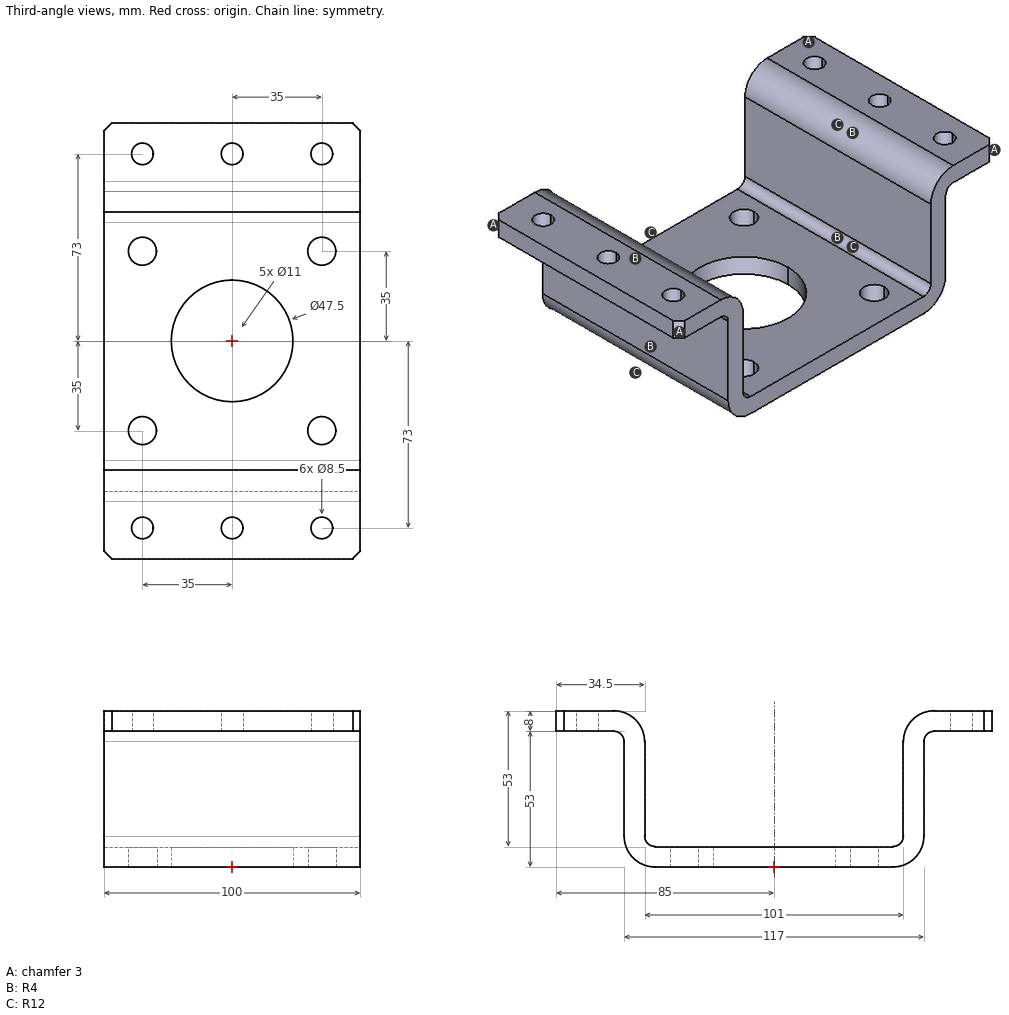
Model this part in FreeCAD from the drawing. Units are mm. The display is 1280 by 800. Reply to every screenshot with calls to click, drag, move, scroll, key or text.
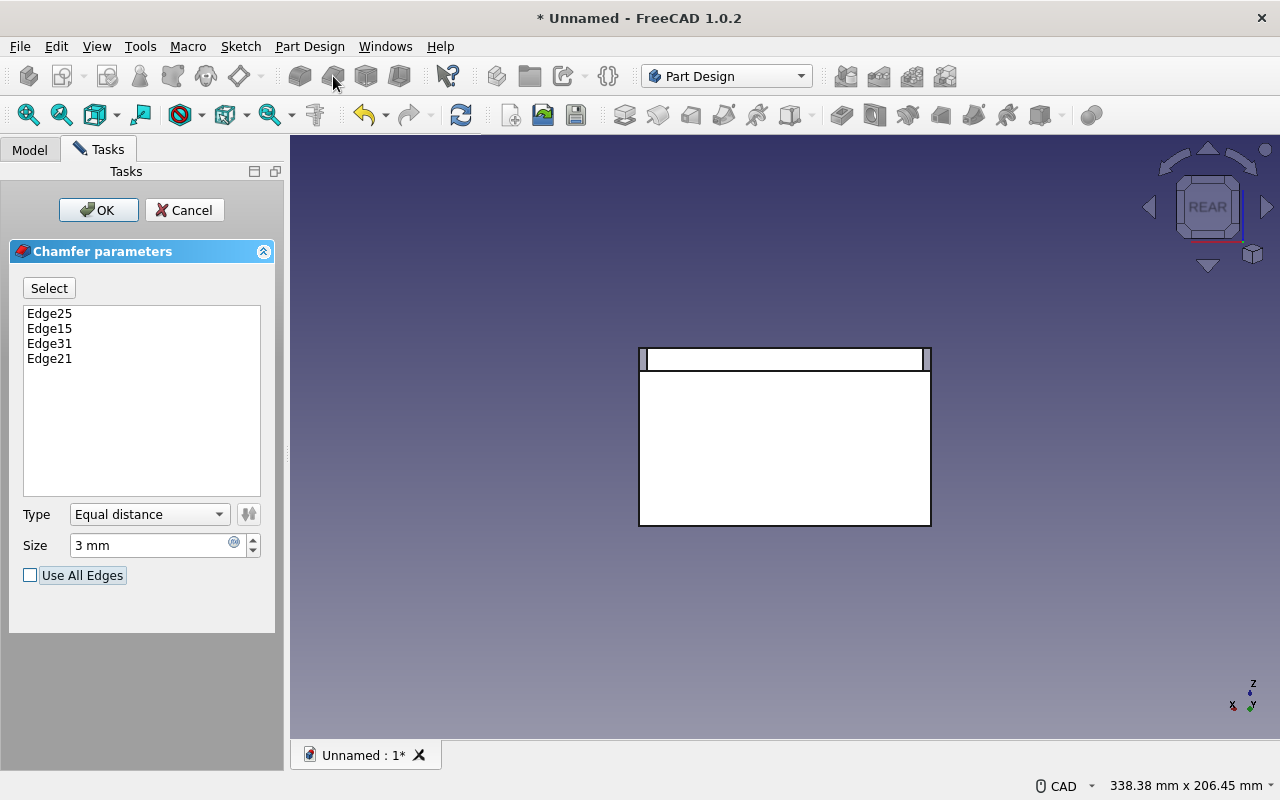
click(99, 210)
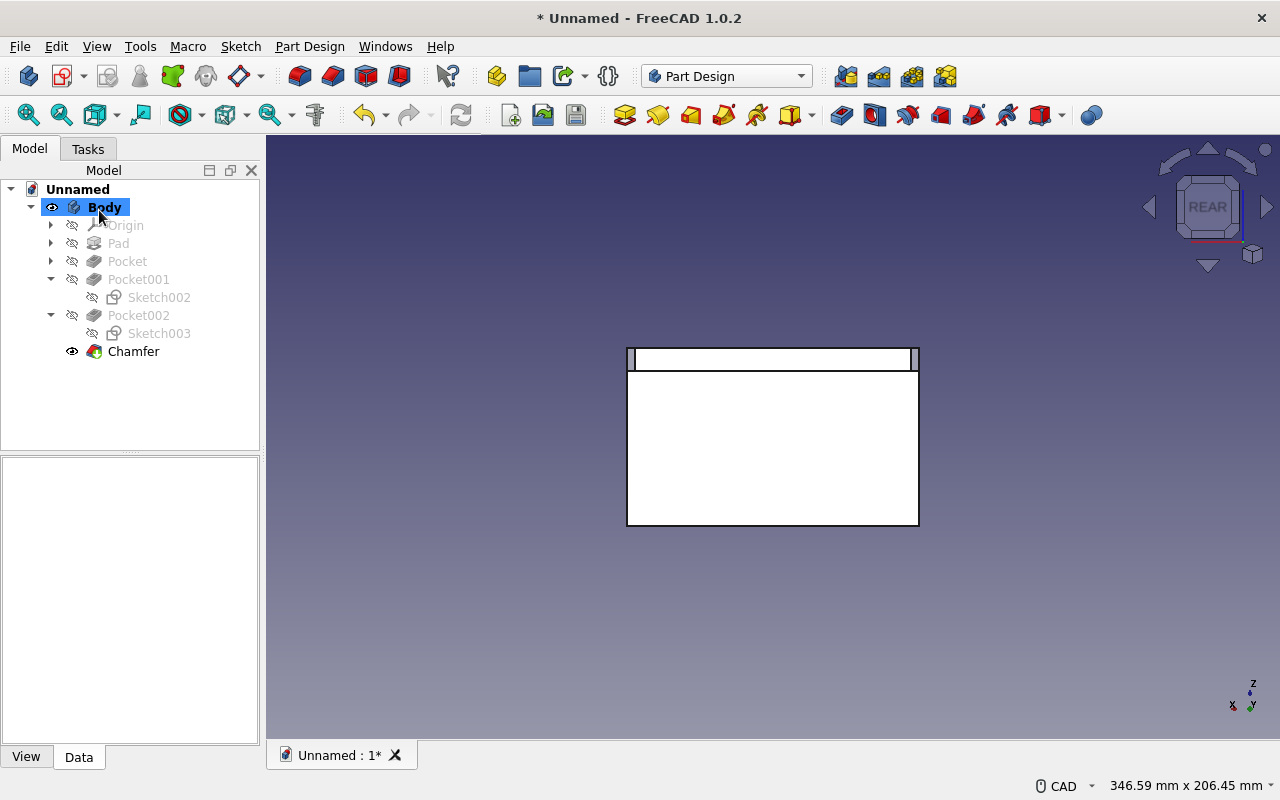
click(29, 116)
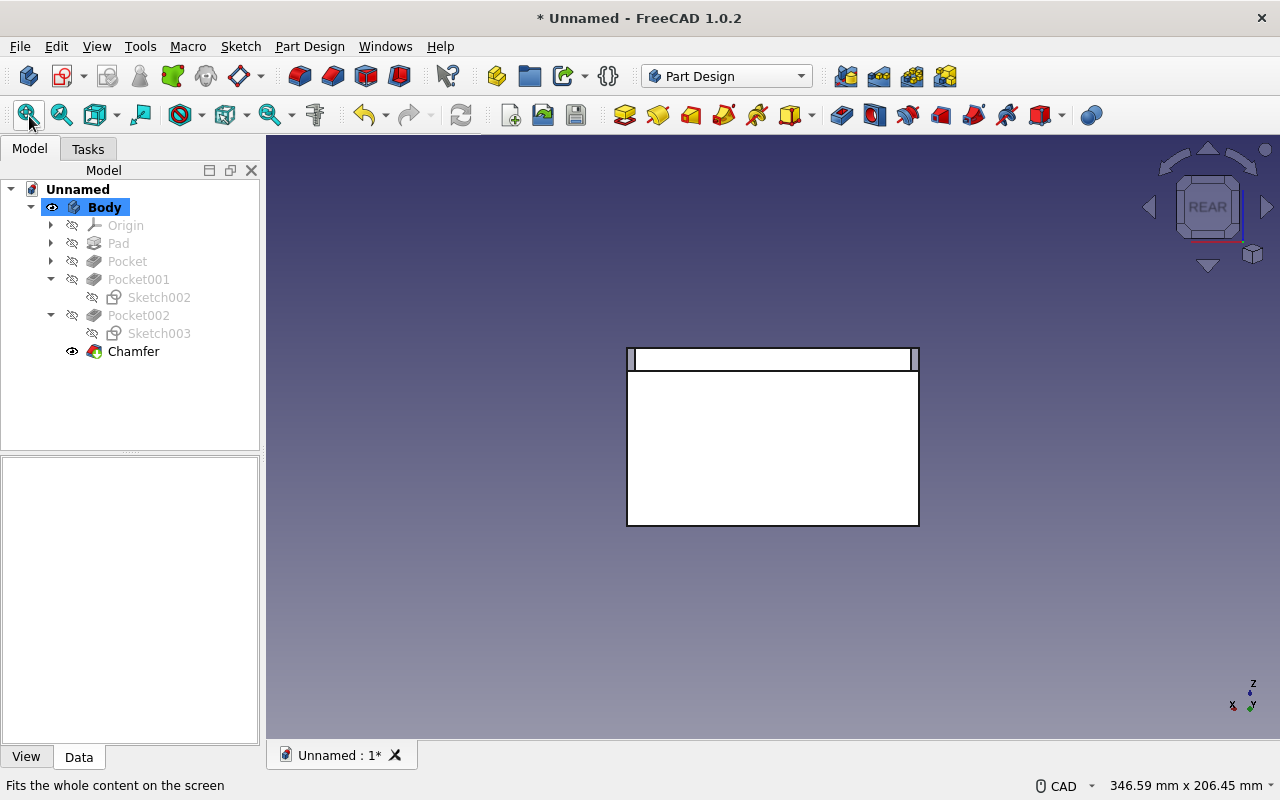
key(0)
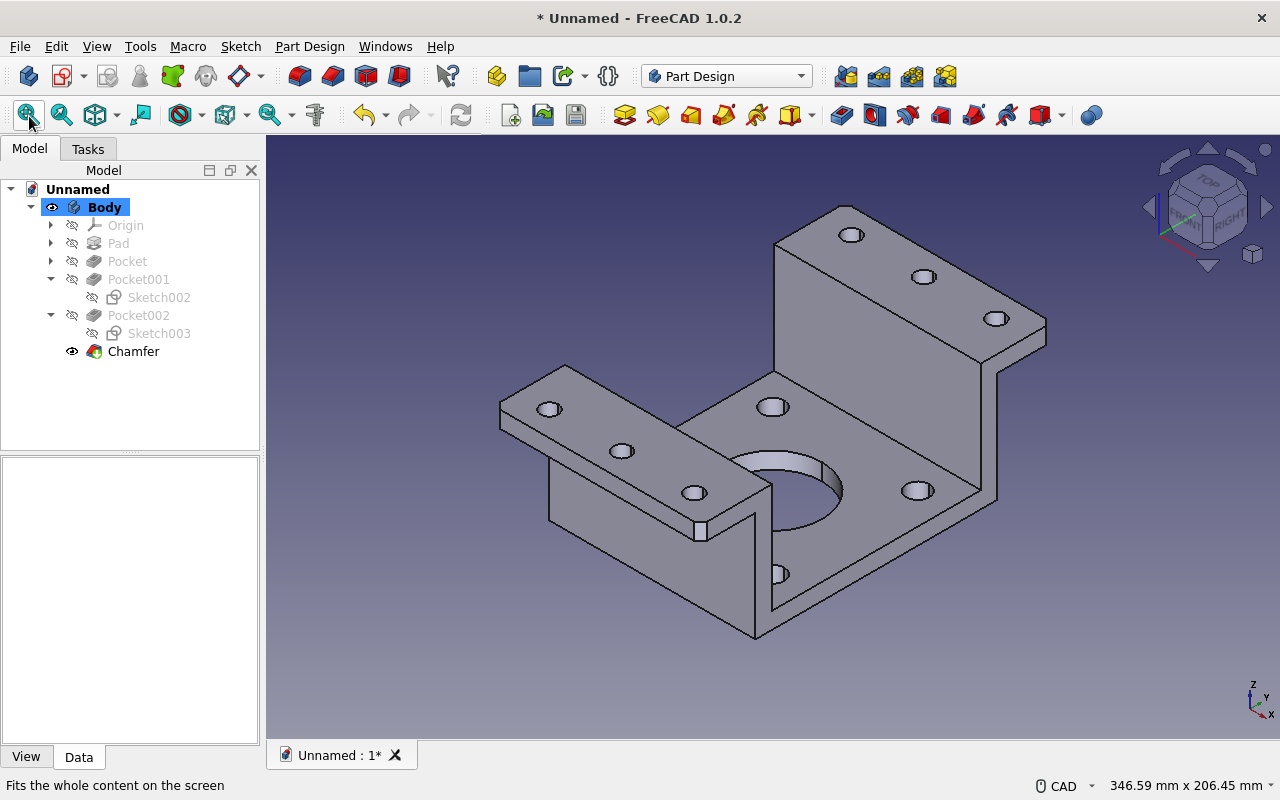
key(2)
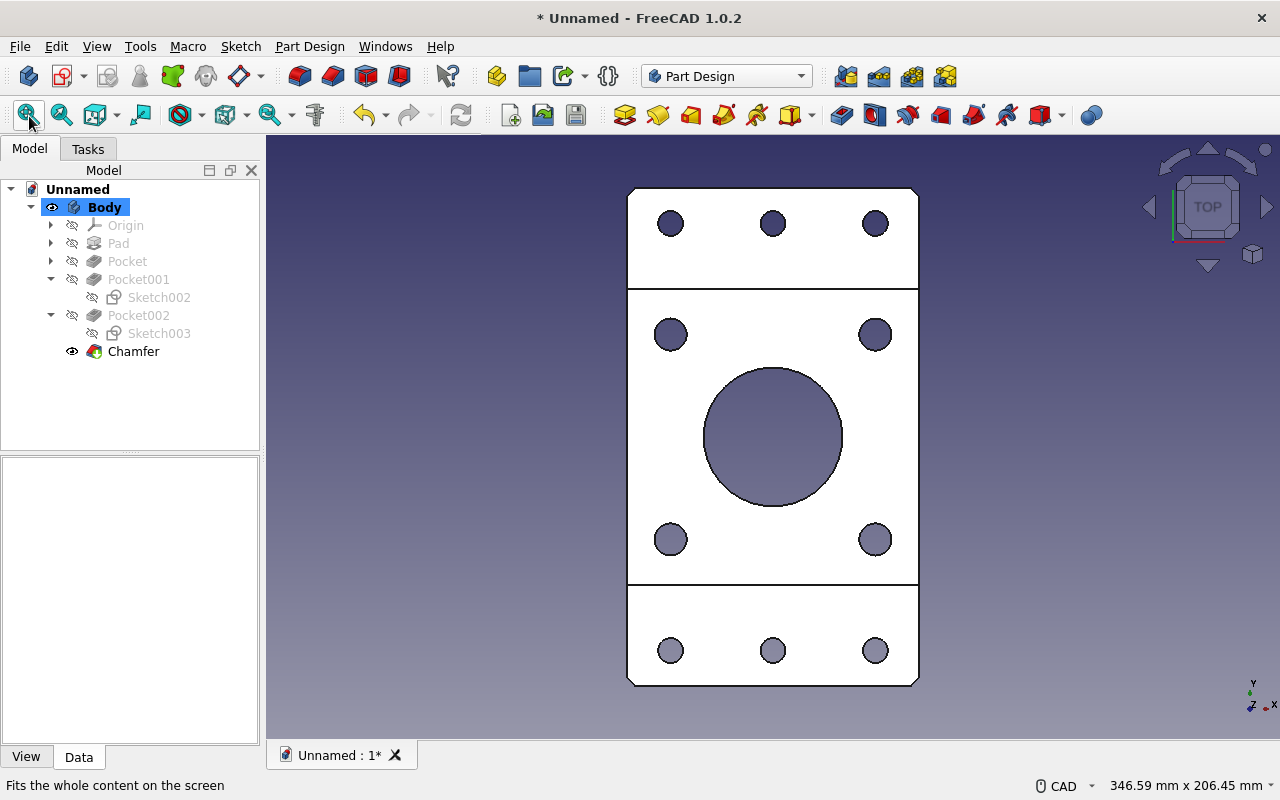
key(1)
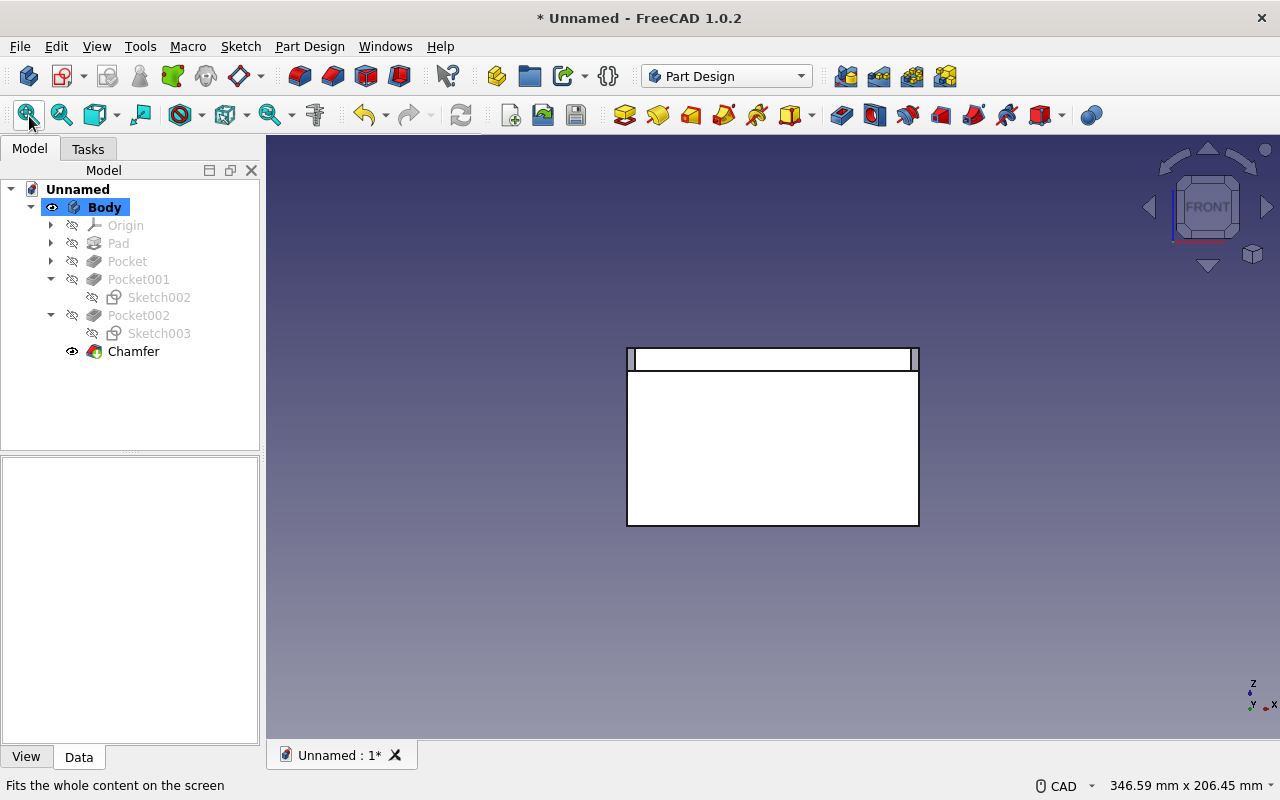
key(v)
key(f)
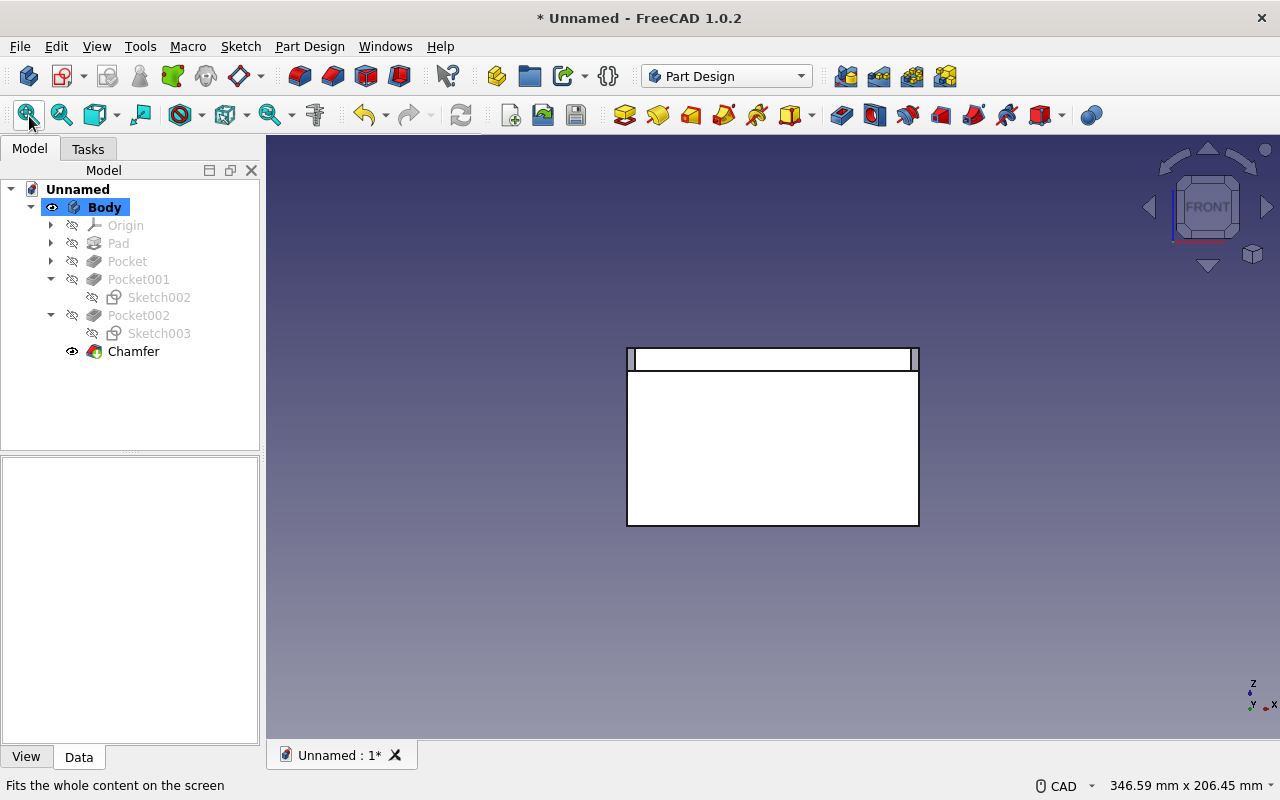
key(3)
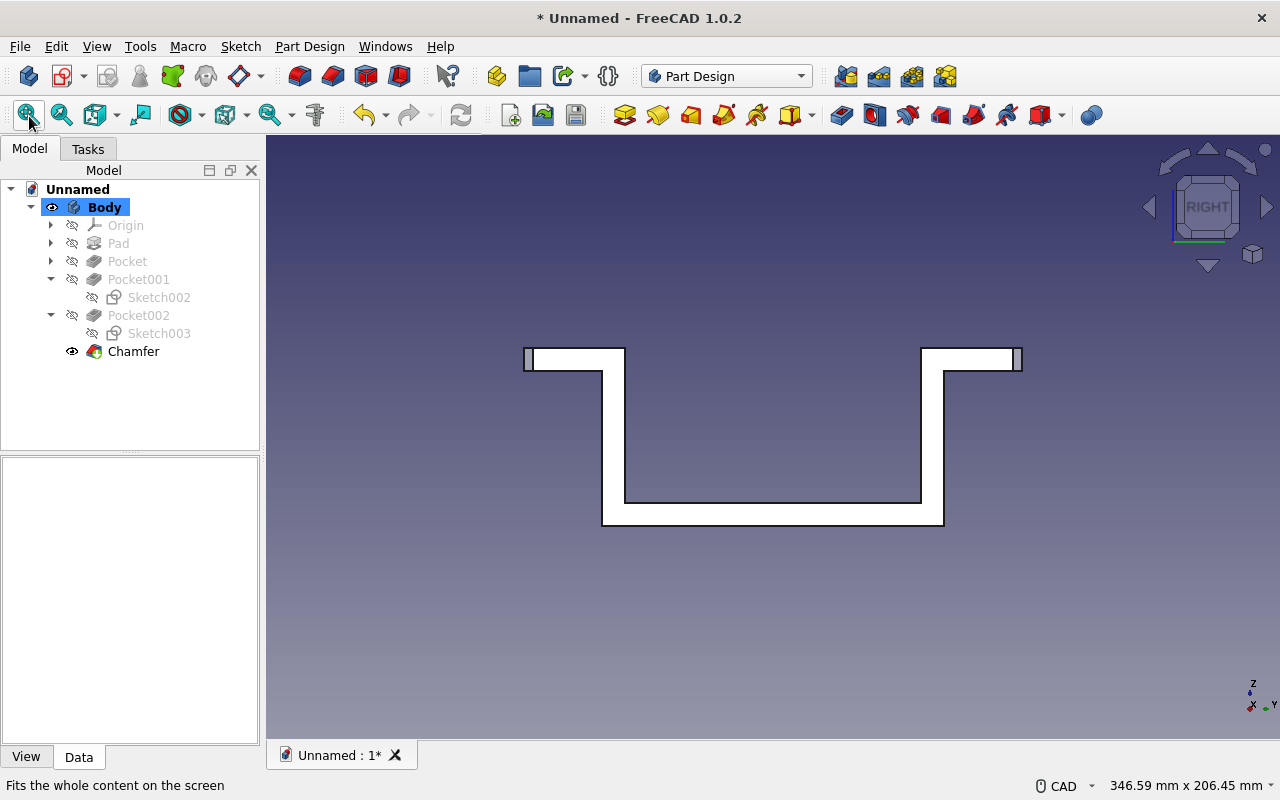
key(5)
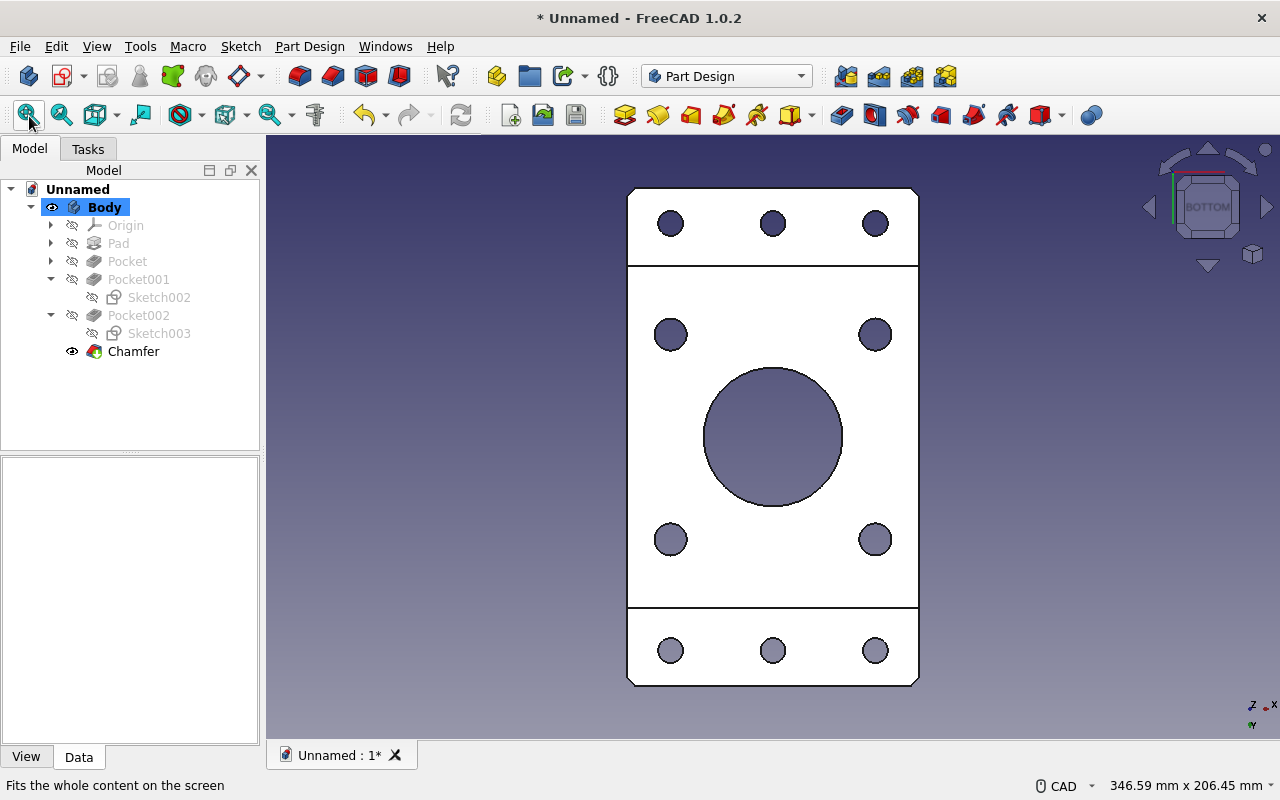
key(4)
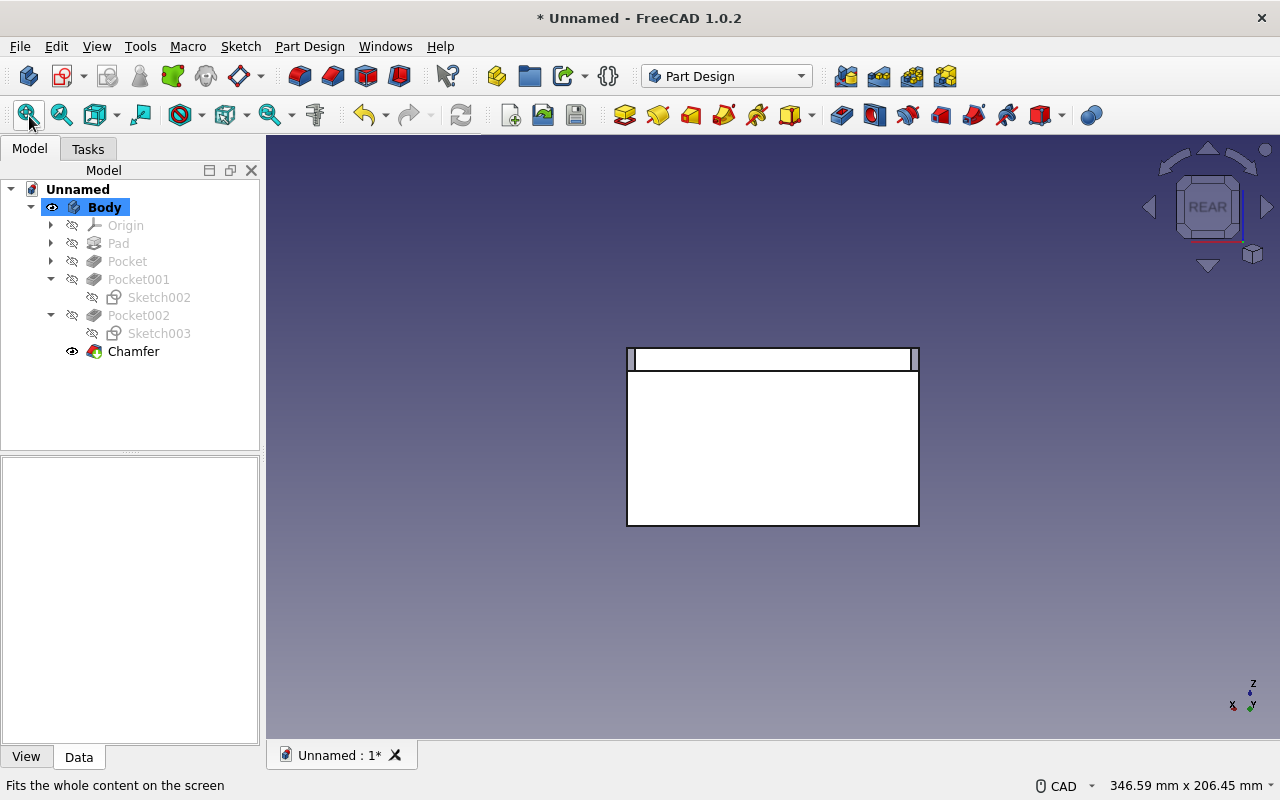
click(29, 116)